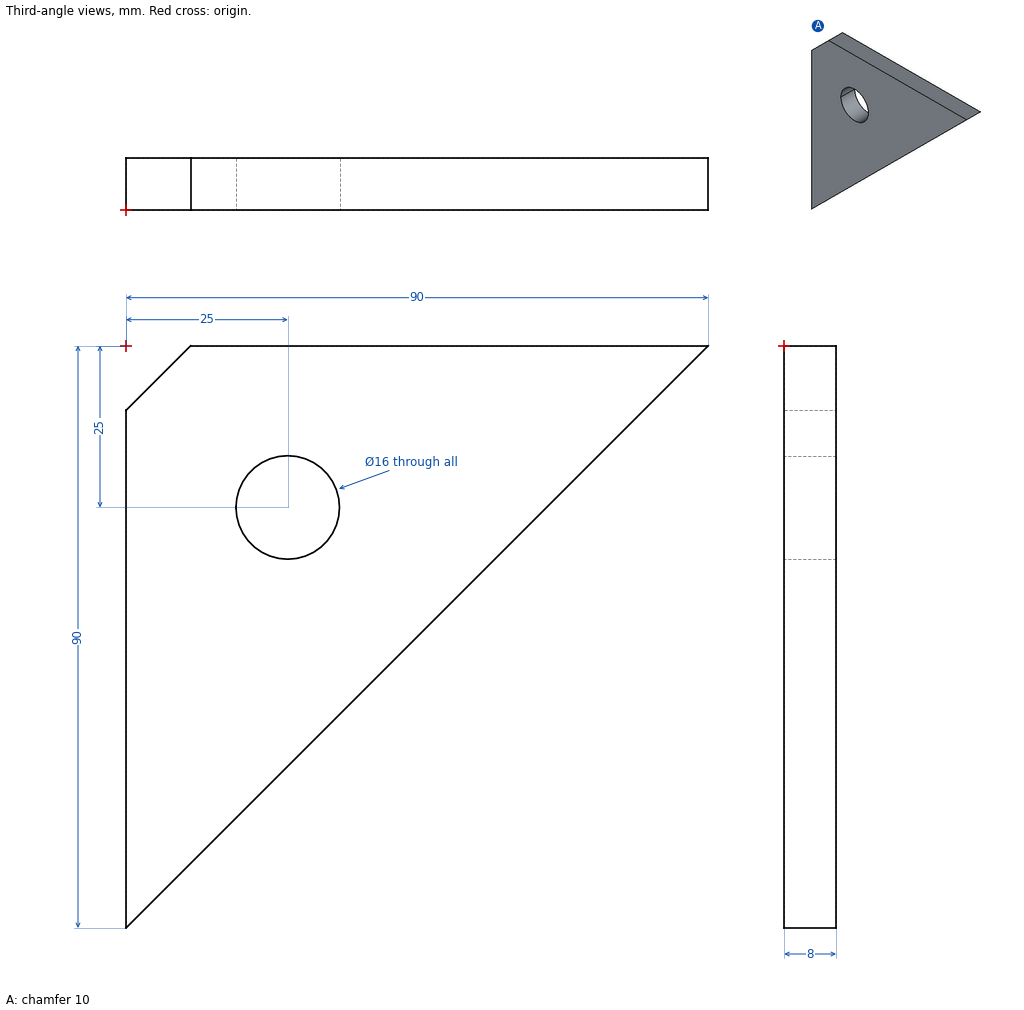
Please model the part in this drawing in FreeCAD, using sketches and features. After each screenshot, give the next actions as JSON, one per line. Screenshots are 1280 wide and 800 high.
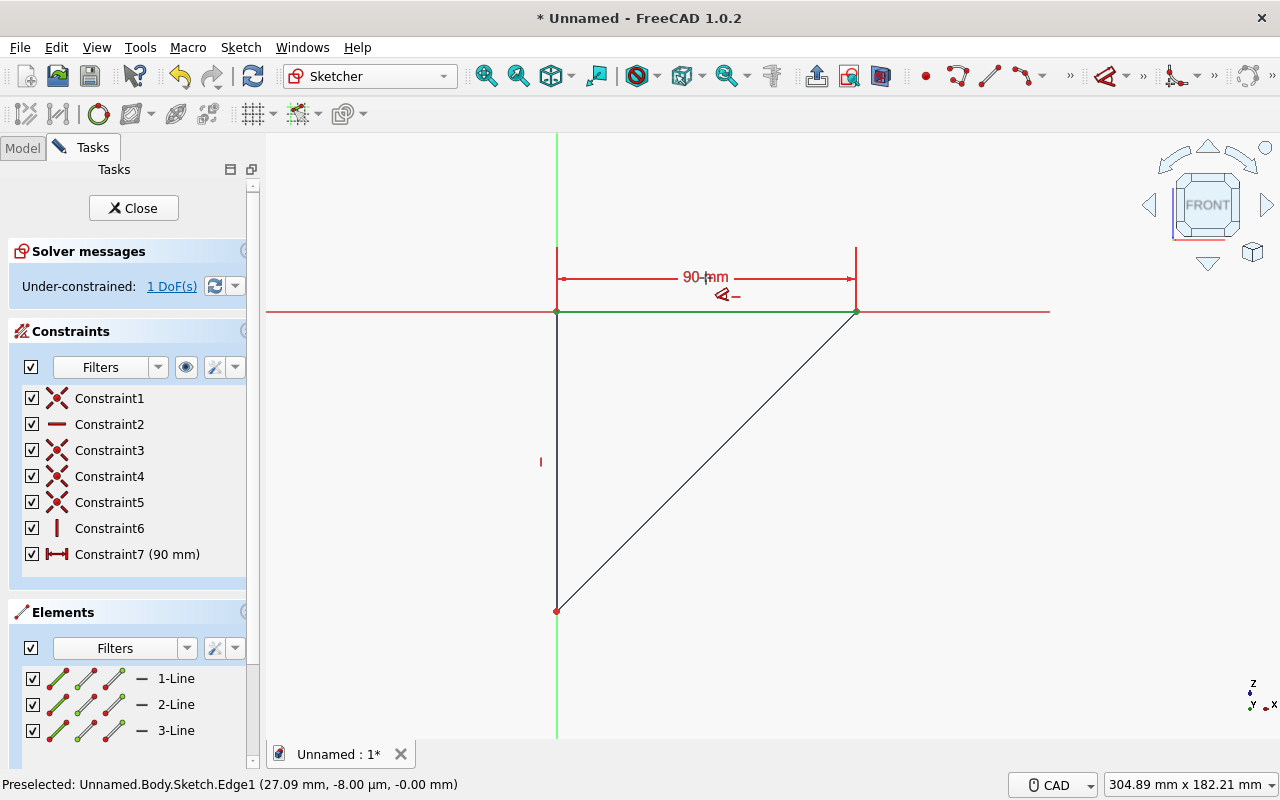
{"action": "left_click", "coordinate": [557, 522]}
{"action": "left_click", "coordinate": [523, 462]}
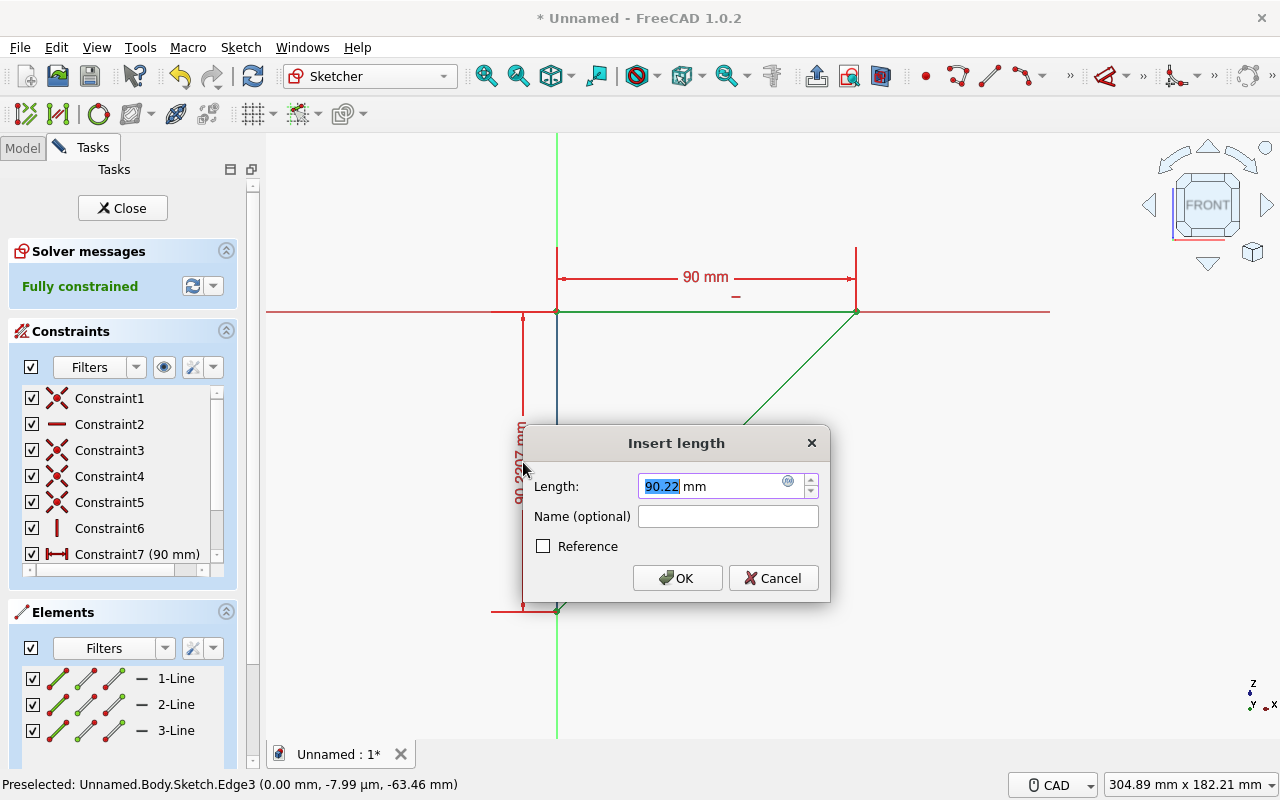
{"action": "type", "text": "90"}
{"action": "key", "text": "Return"}
{"action": "key", "text": "Escape"}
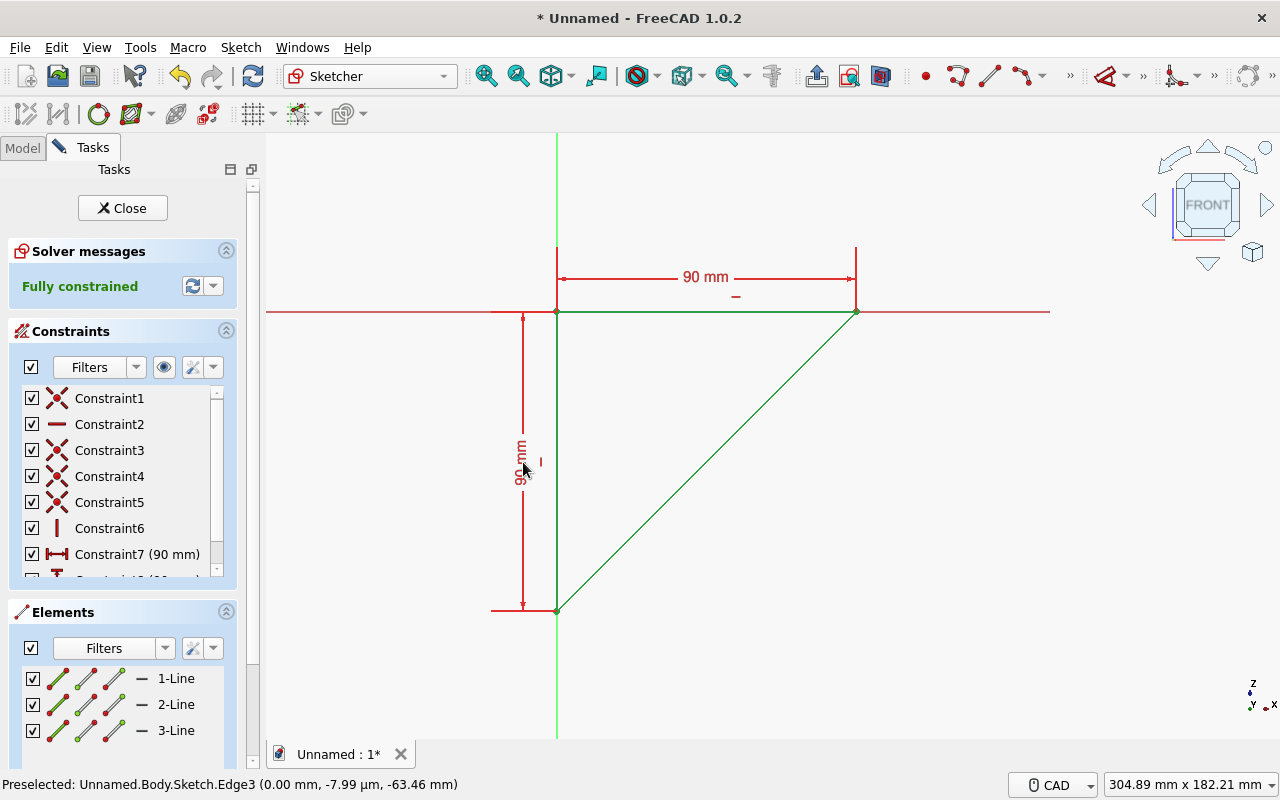
{"action": "left_click", "coordinate": [123, 208]}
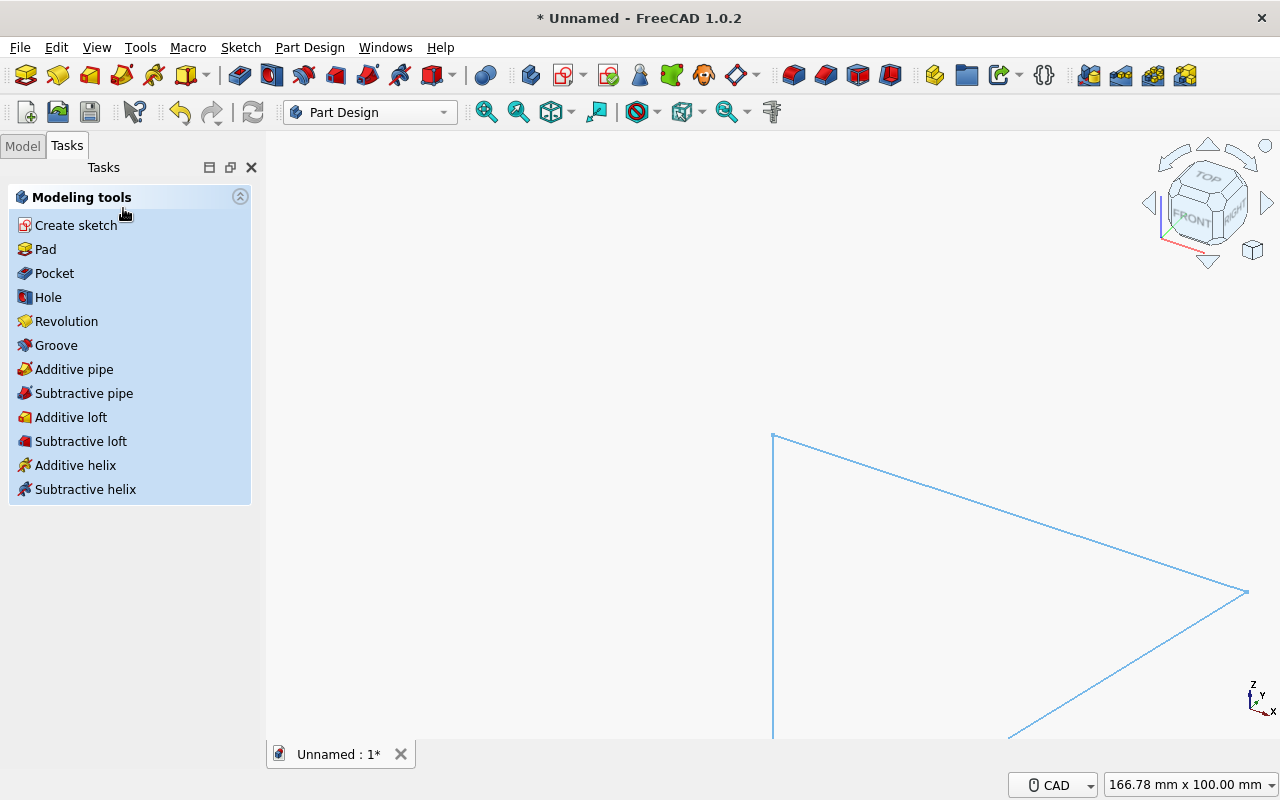
{"action": "left_click", "coordinate": [26, 76]}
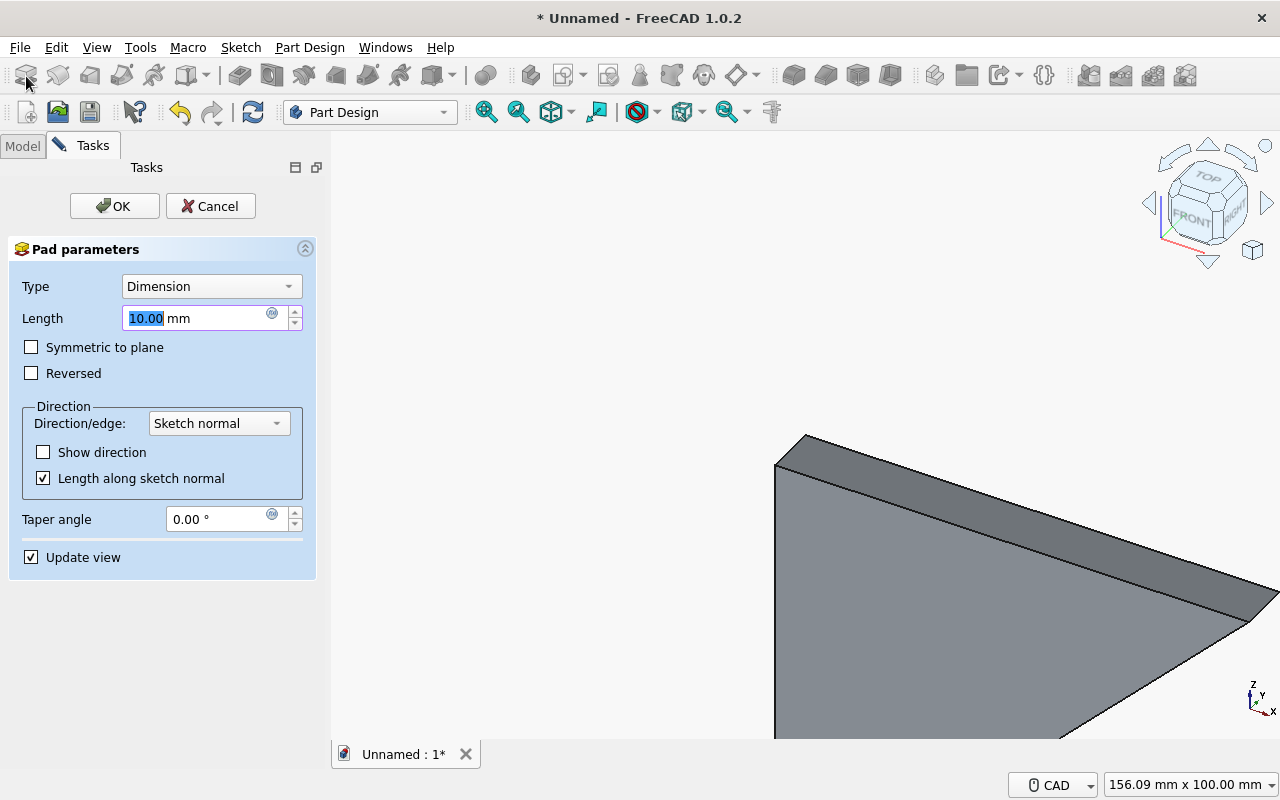
{"action": "type", "text": "8"}
{"action": "key", "text": "Tab"}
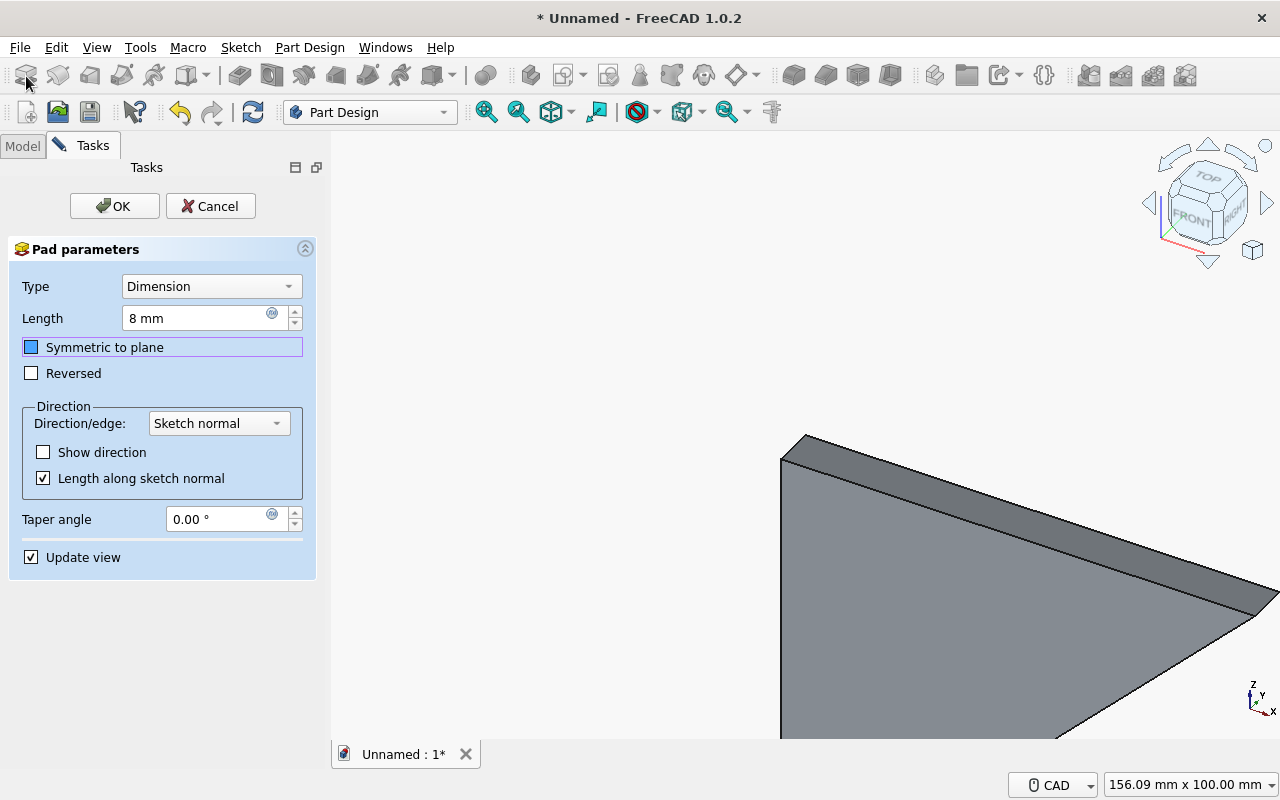
{"action": "left_click", "coordinate": [30, 373]}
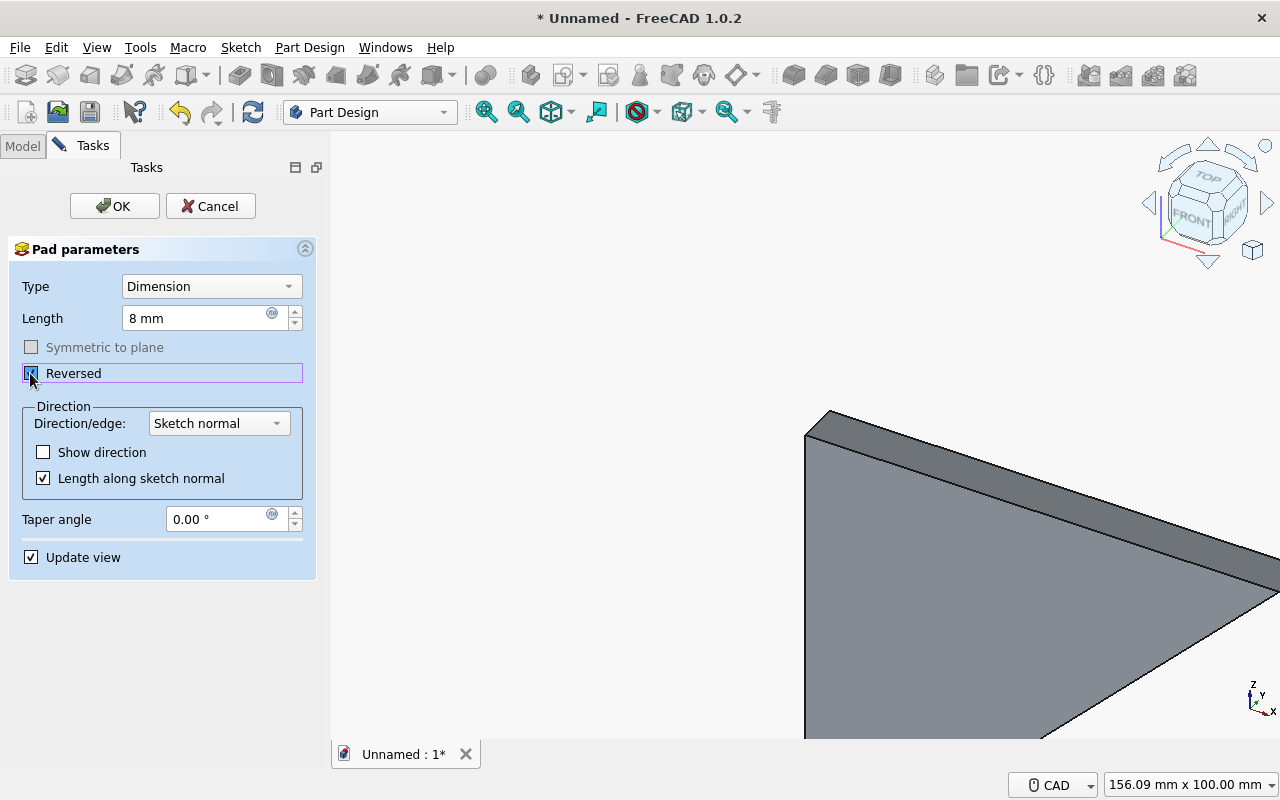
{"action": "left_click", "coordinate": [115, 206]}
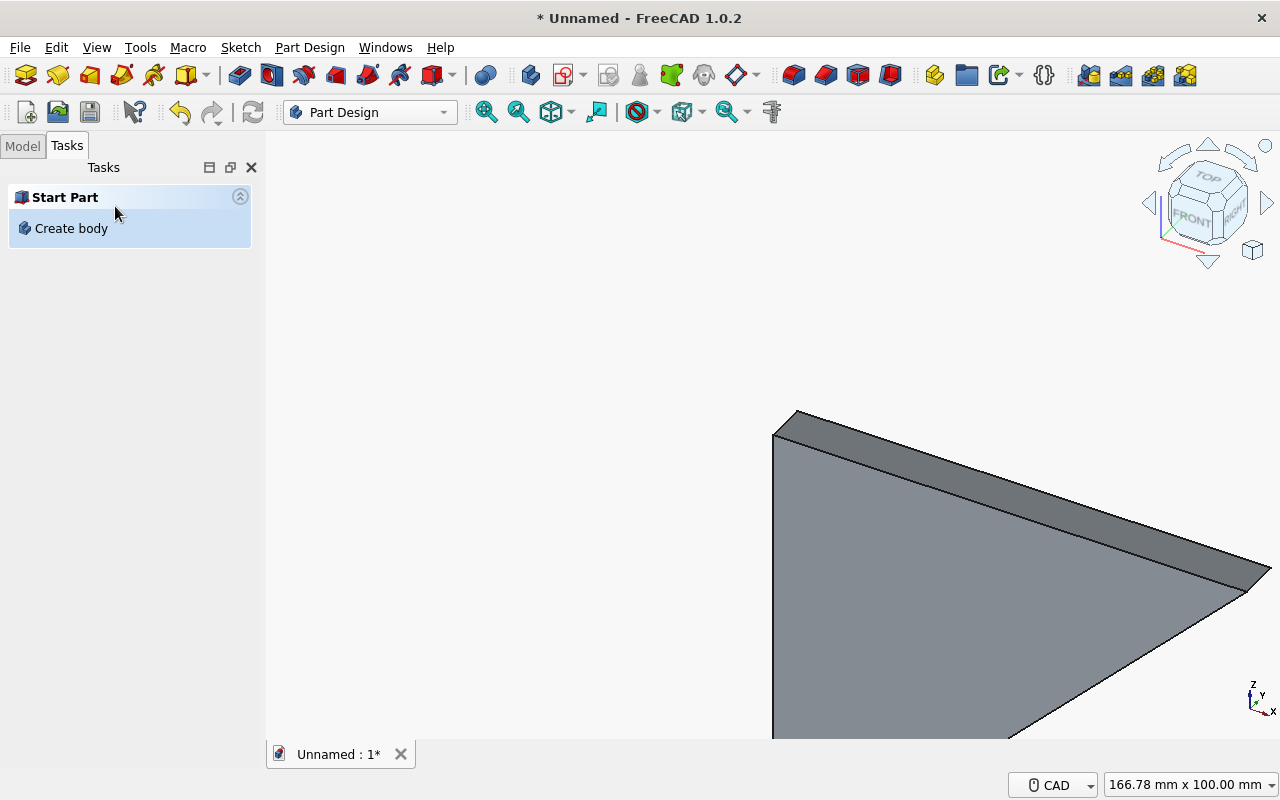
{"action": "left_click", "coordinate": [488, 112]}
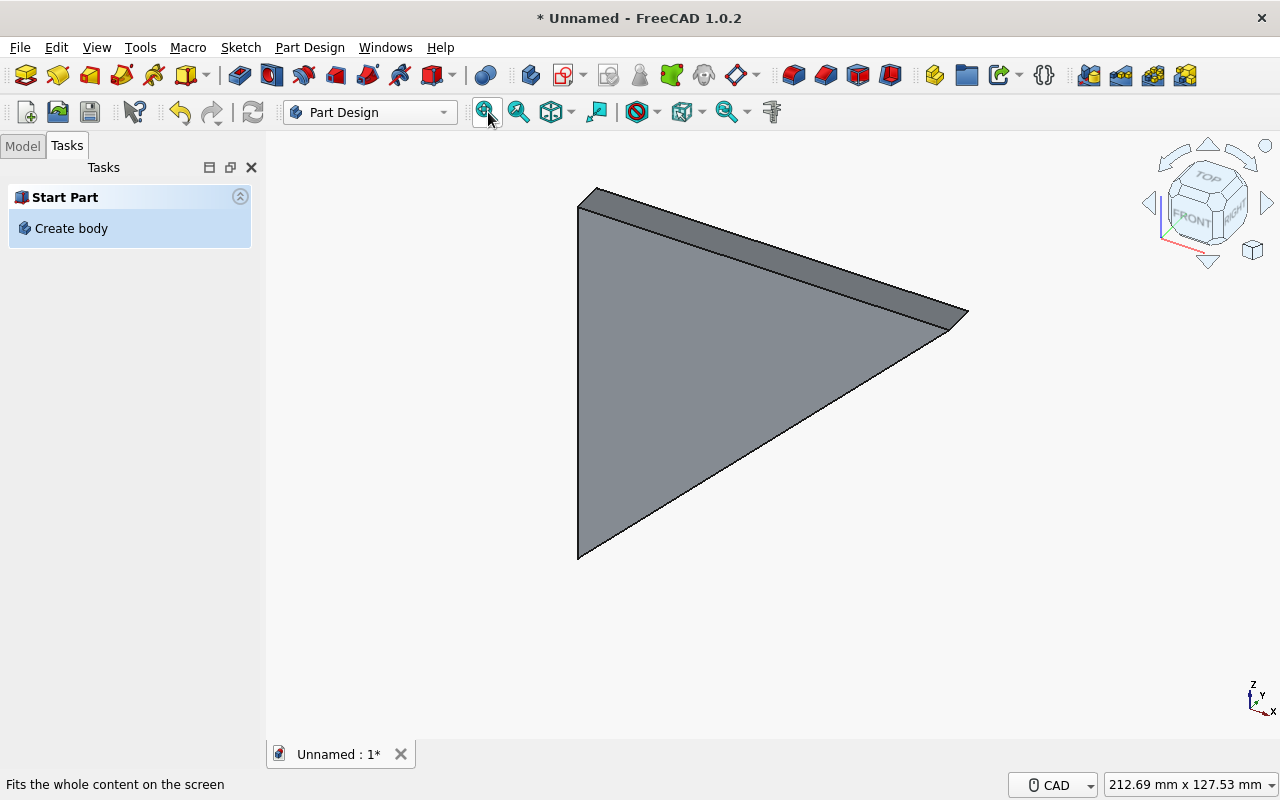
{"action": "key", "text": "0"}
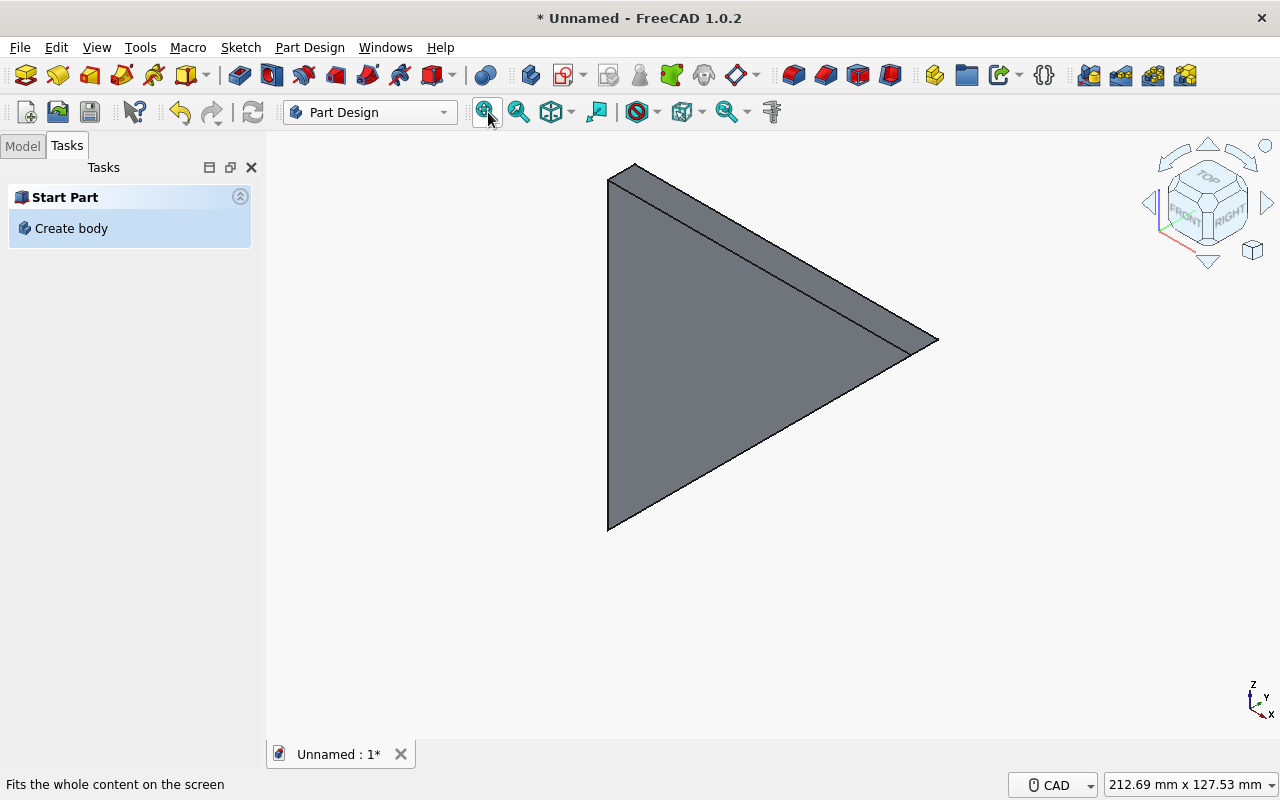
{"action": "key", "text": "2"}